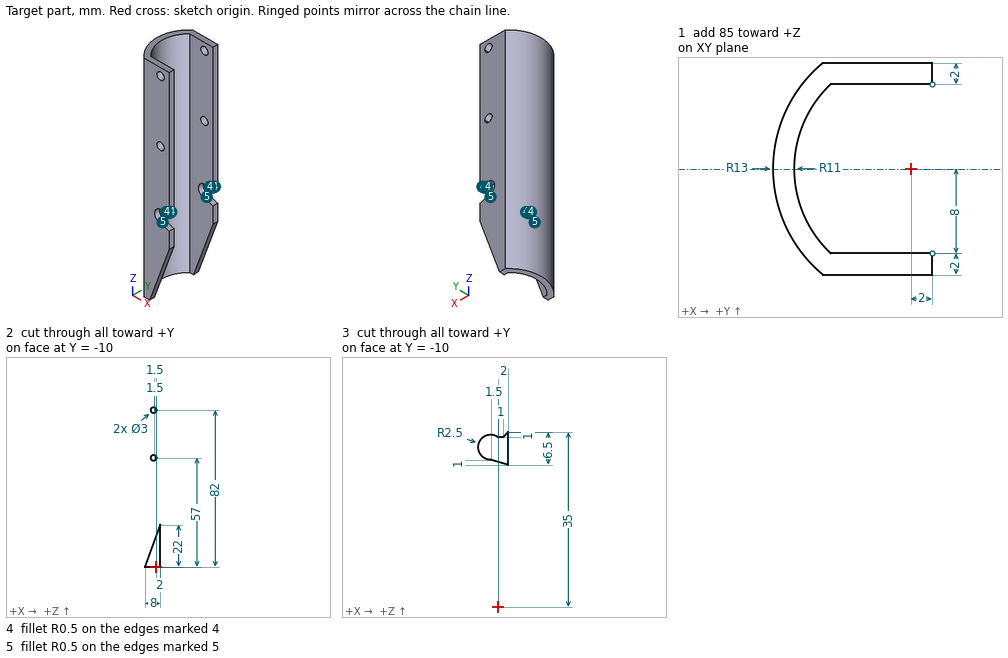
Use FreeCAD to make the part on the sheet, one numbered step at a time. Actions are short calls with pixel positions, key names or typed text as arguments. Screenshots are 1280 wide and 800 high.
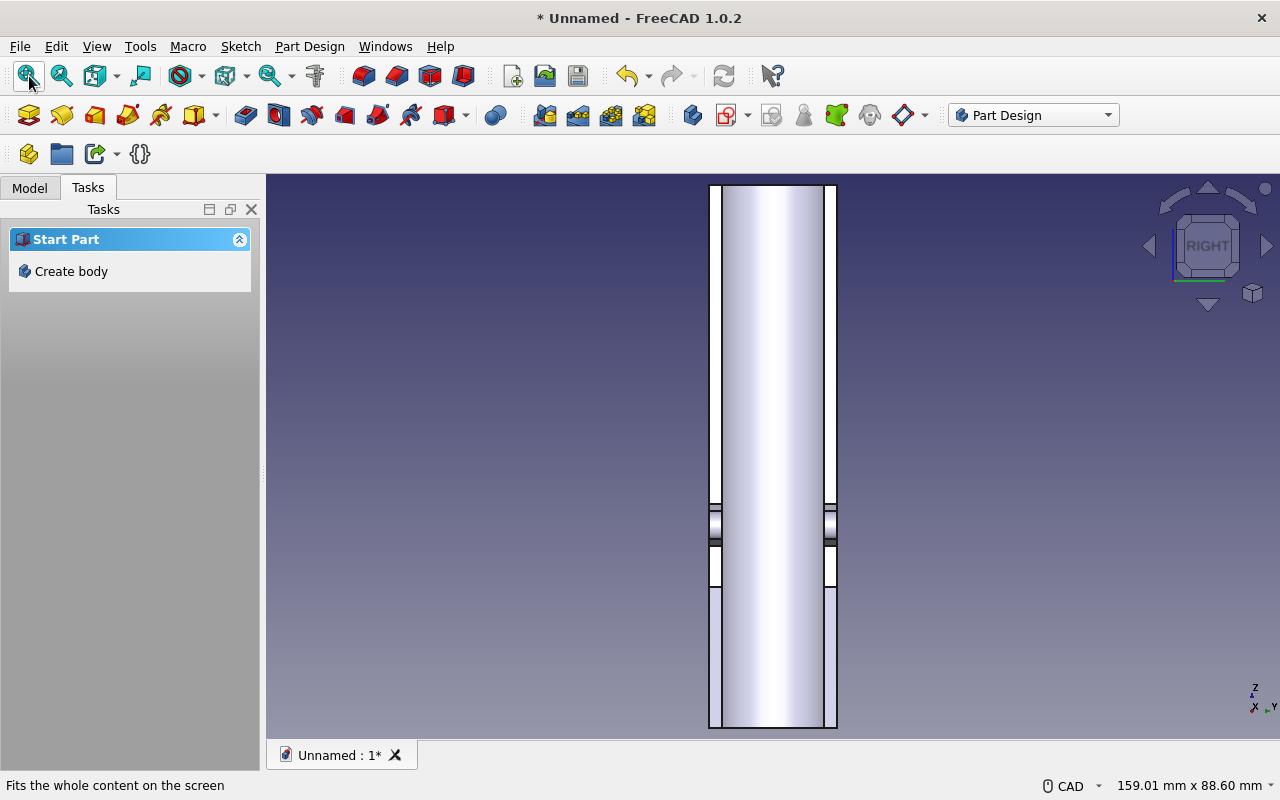
click(716, 503)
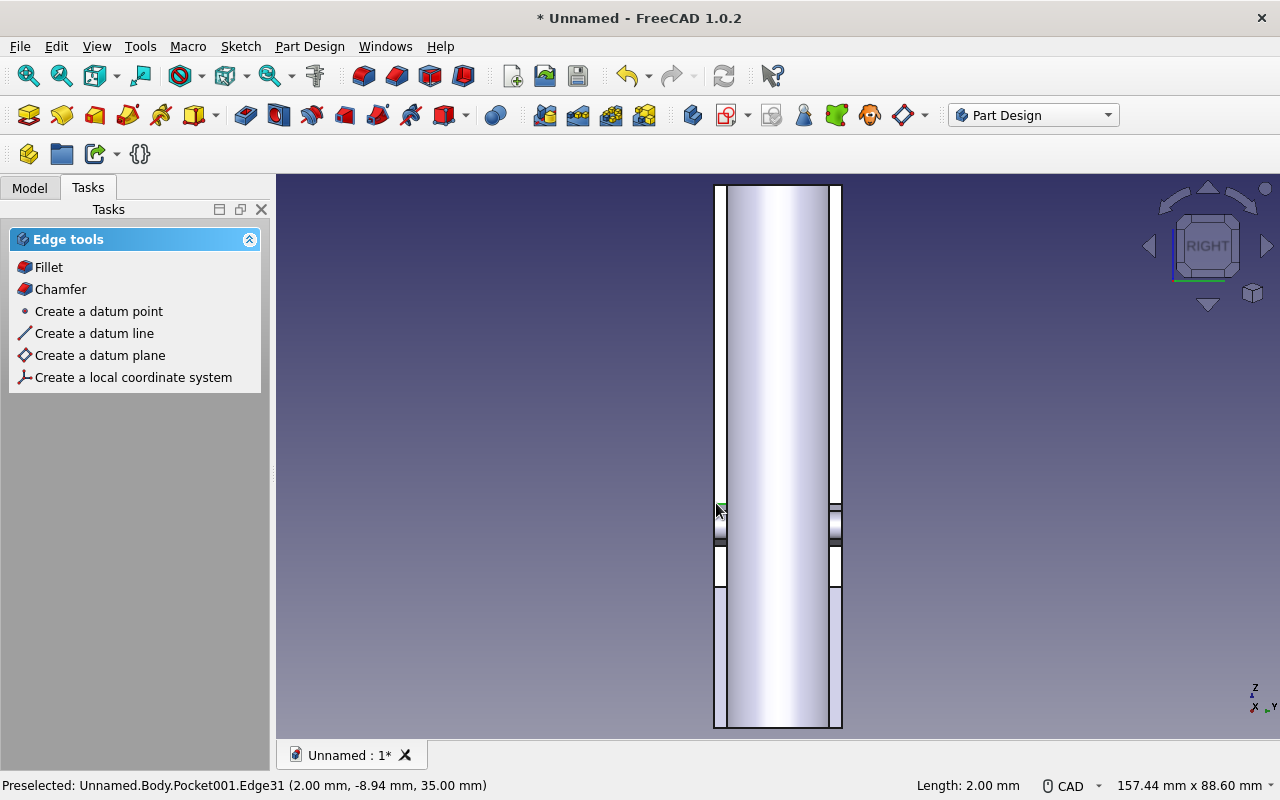
scroll(721, 510, up, 6)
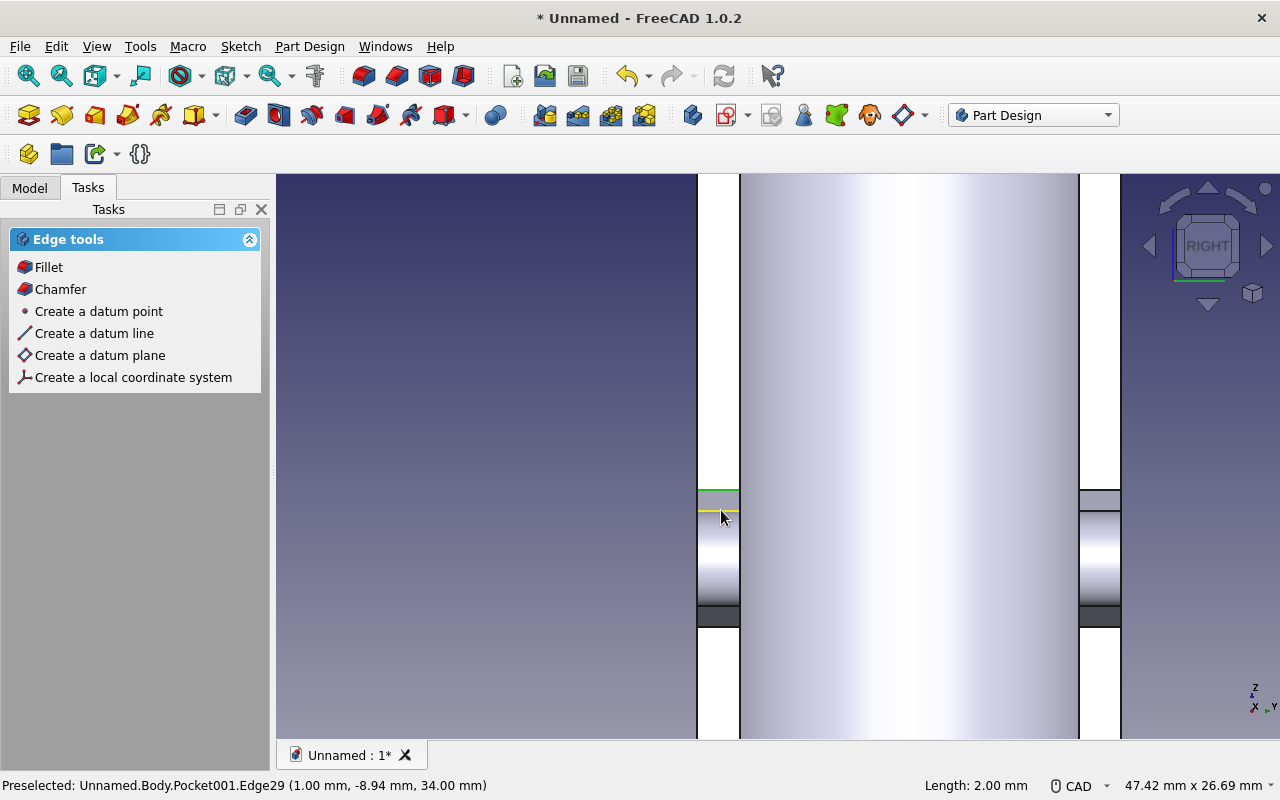
click(1100, 489, ctrl)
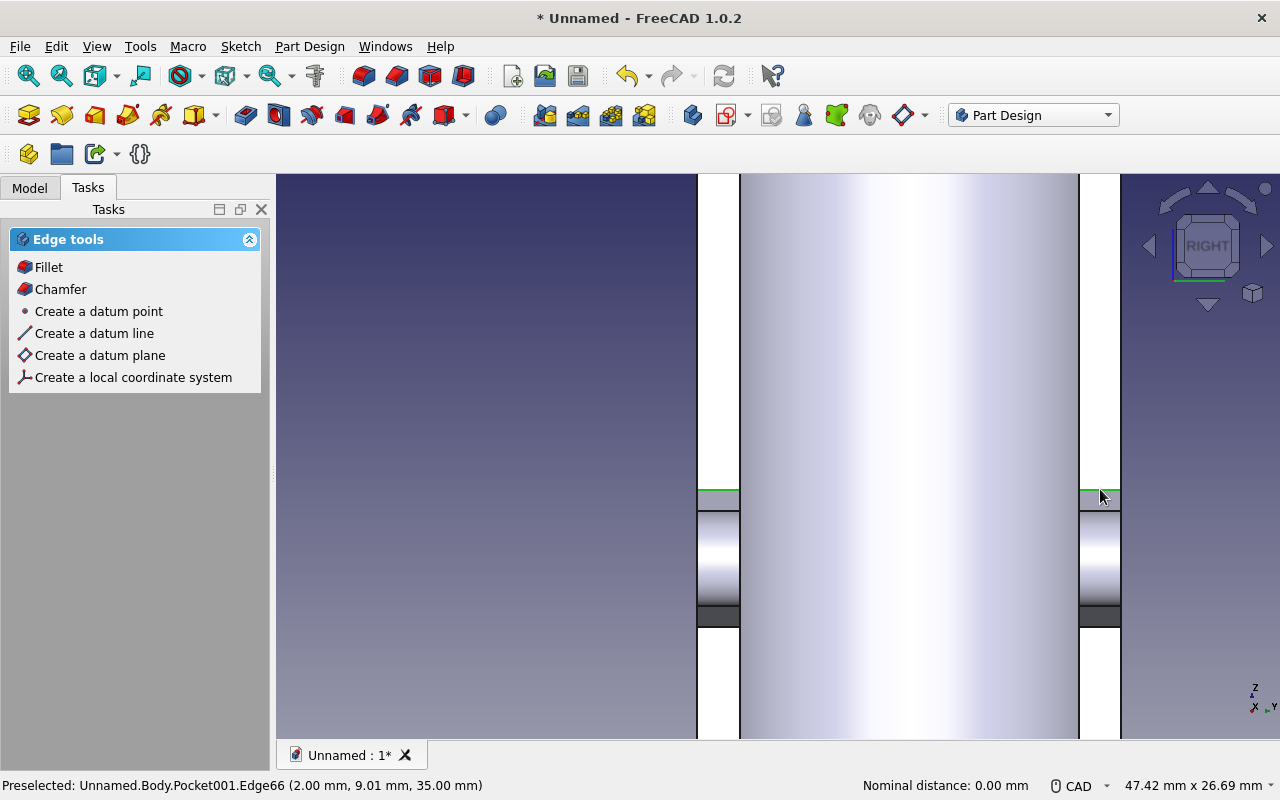
click(29, 76)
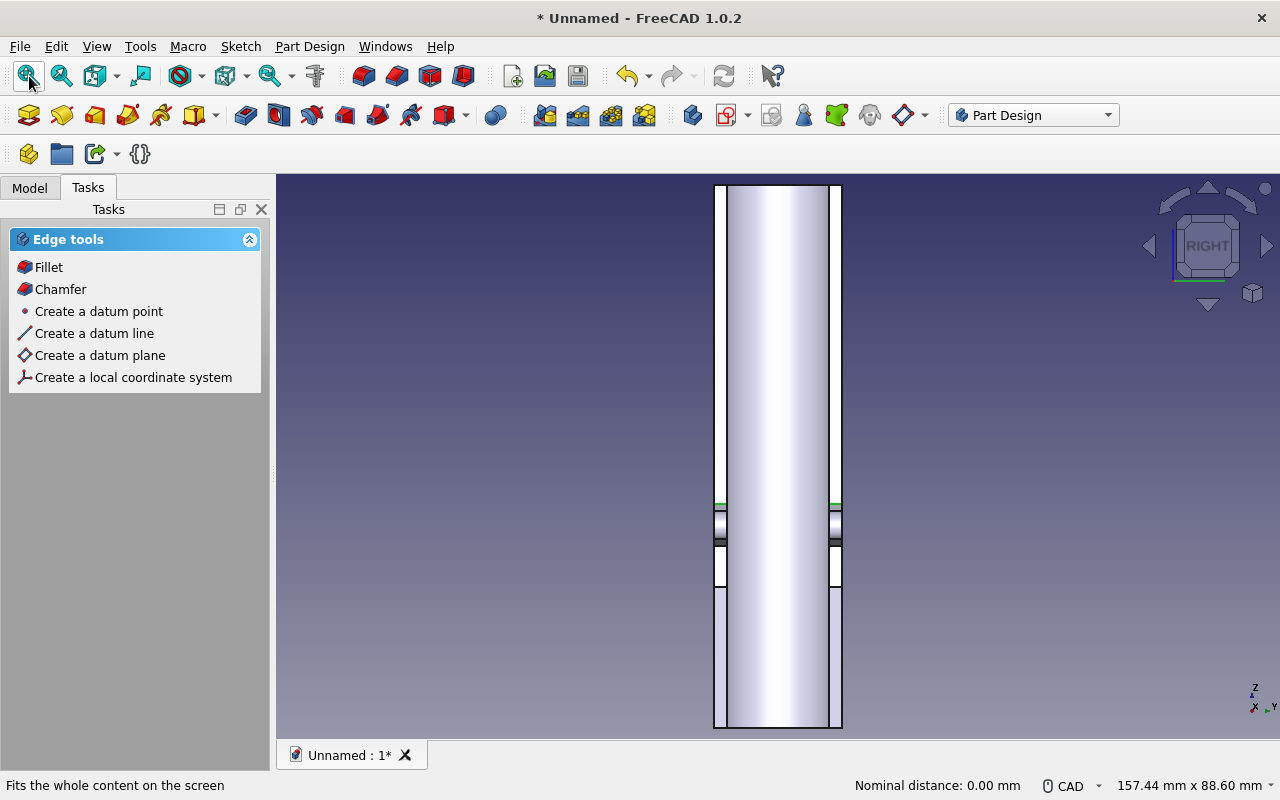
key(5)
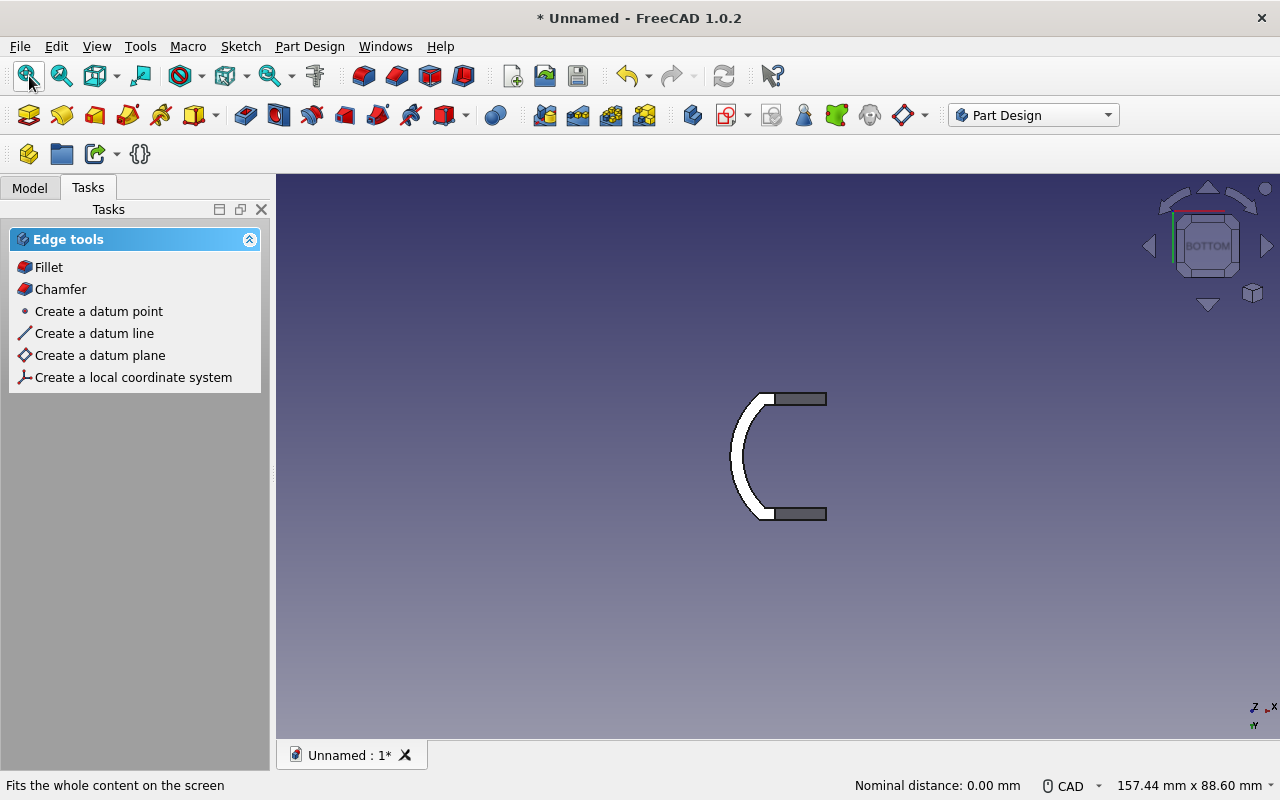
key(v)
key(f)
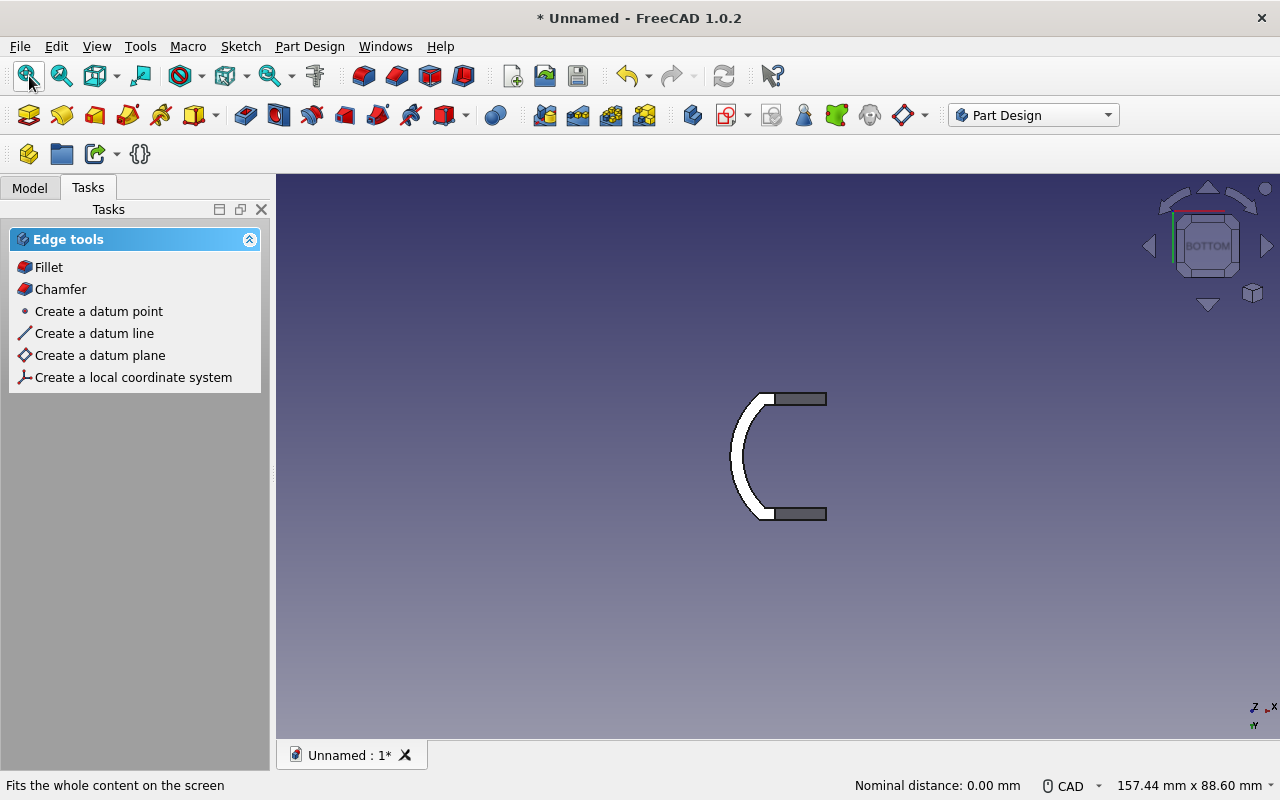
scroll(819, 398, up, 6)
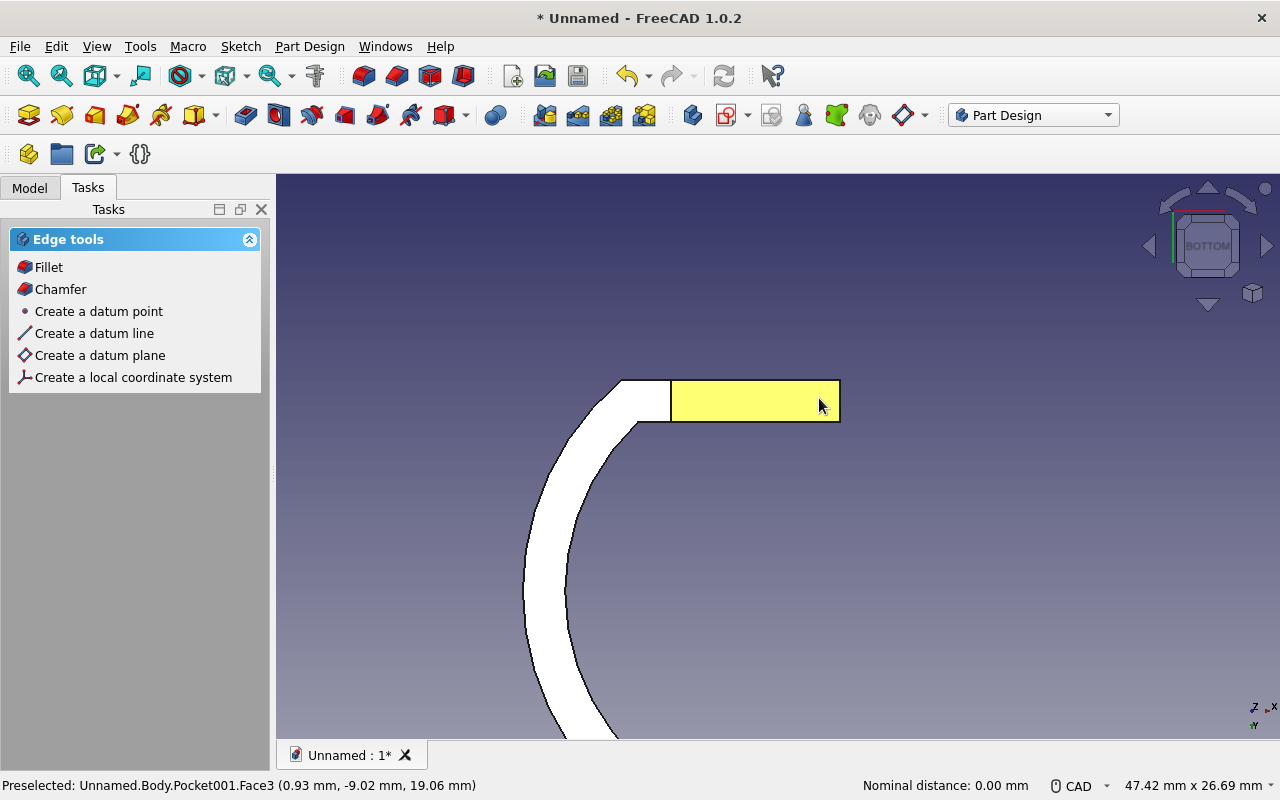
click(29, 76)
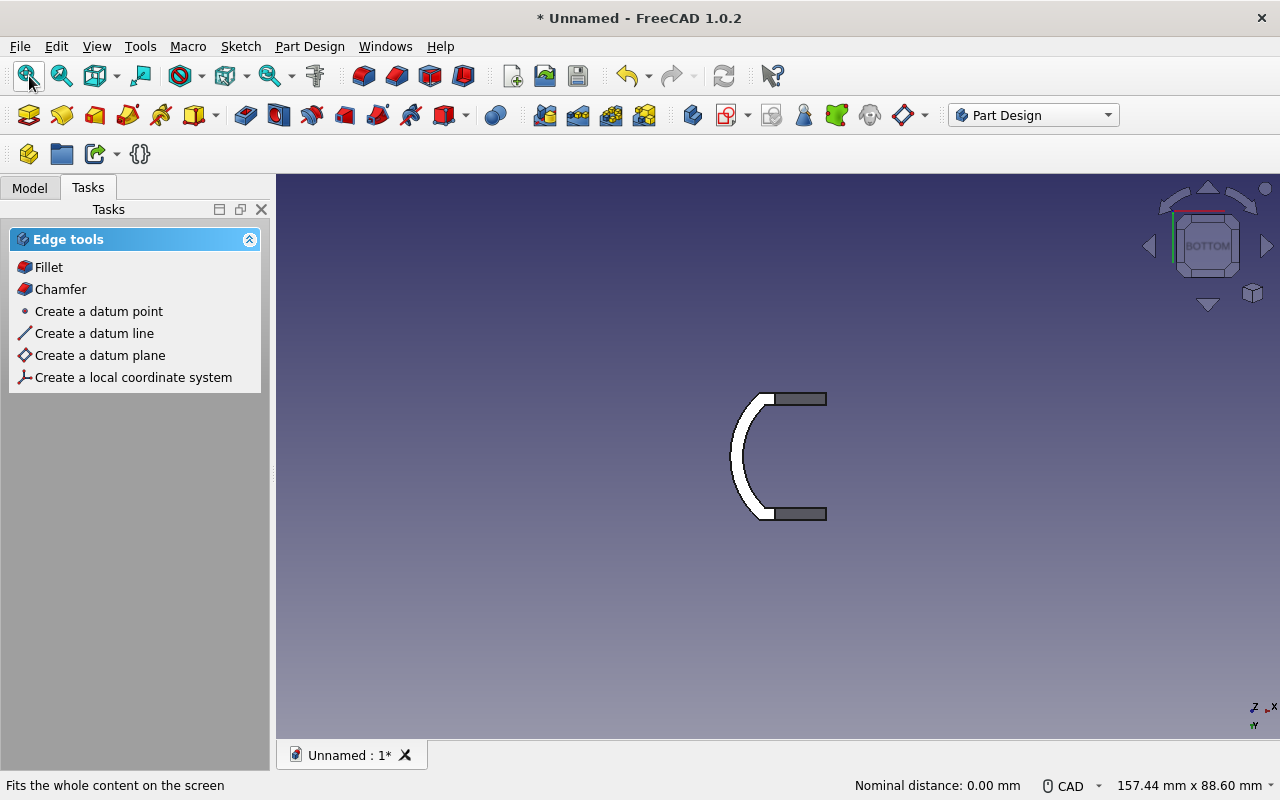
key(4)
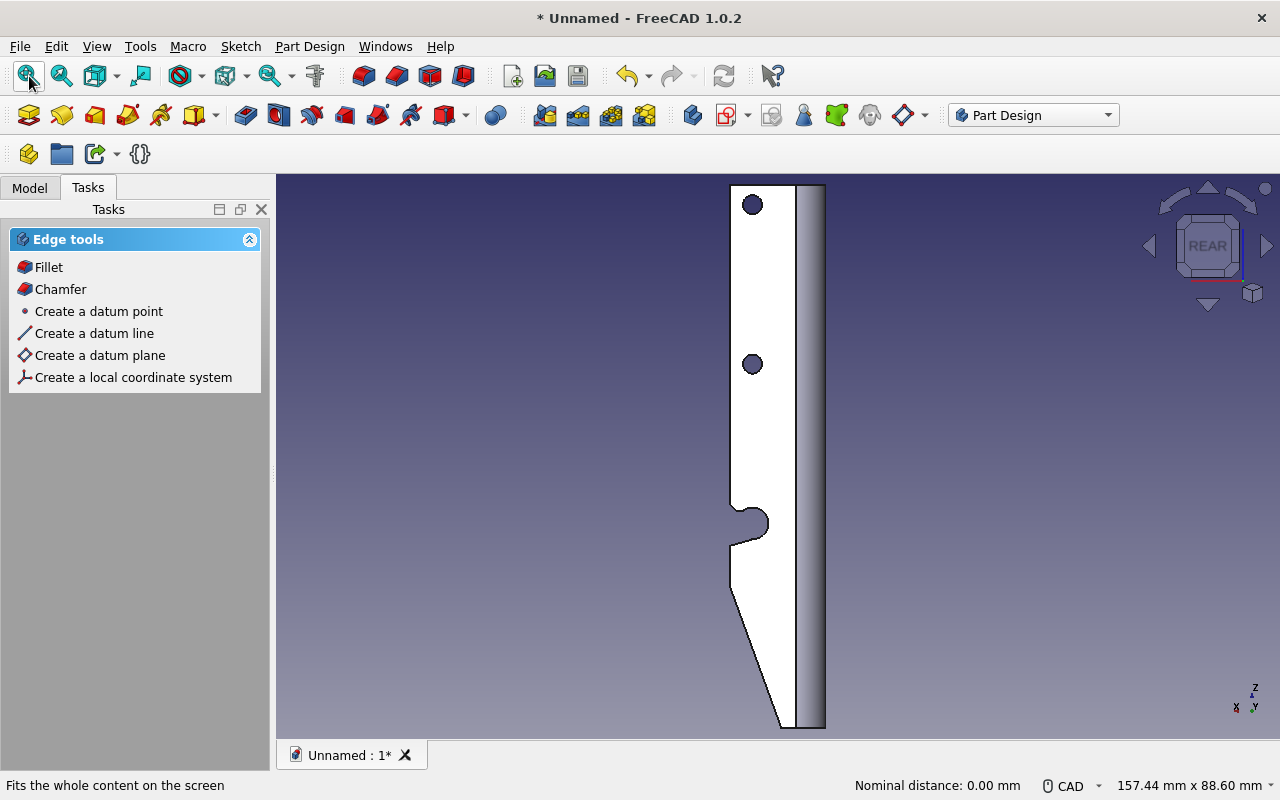
scroll(737, 510, up, 6)